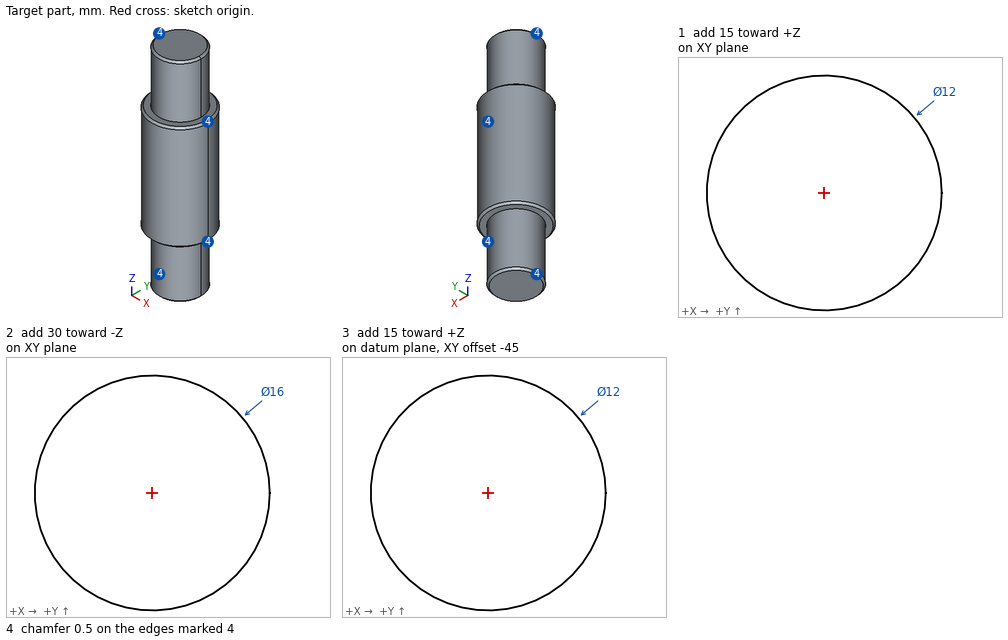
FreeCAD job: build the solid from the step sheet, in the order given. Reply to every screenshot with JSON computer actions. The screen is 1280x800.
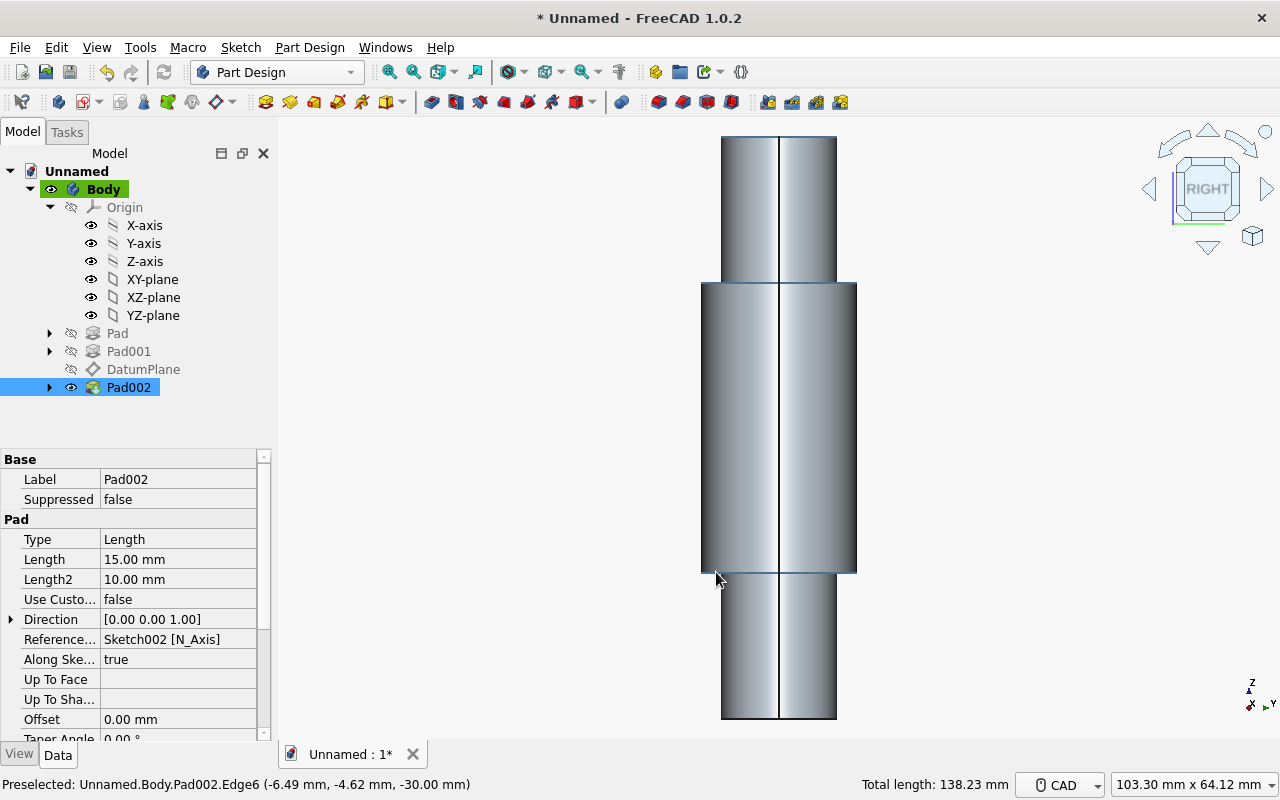
{"action": "key", "text": "5"}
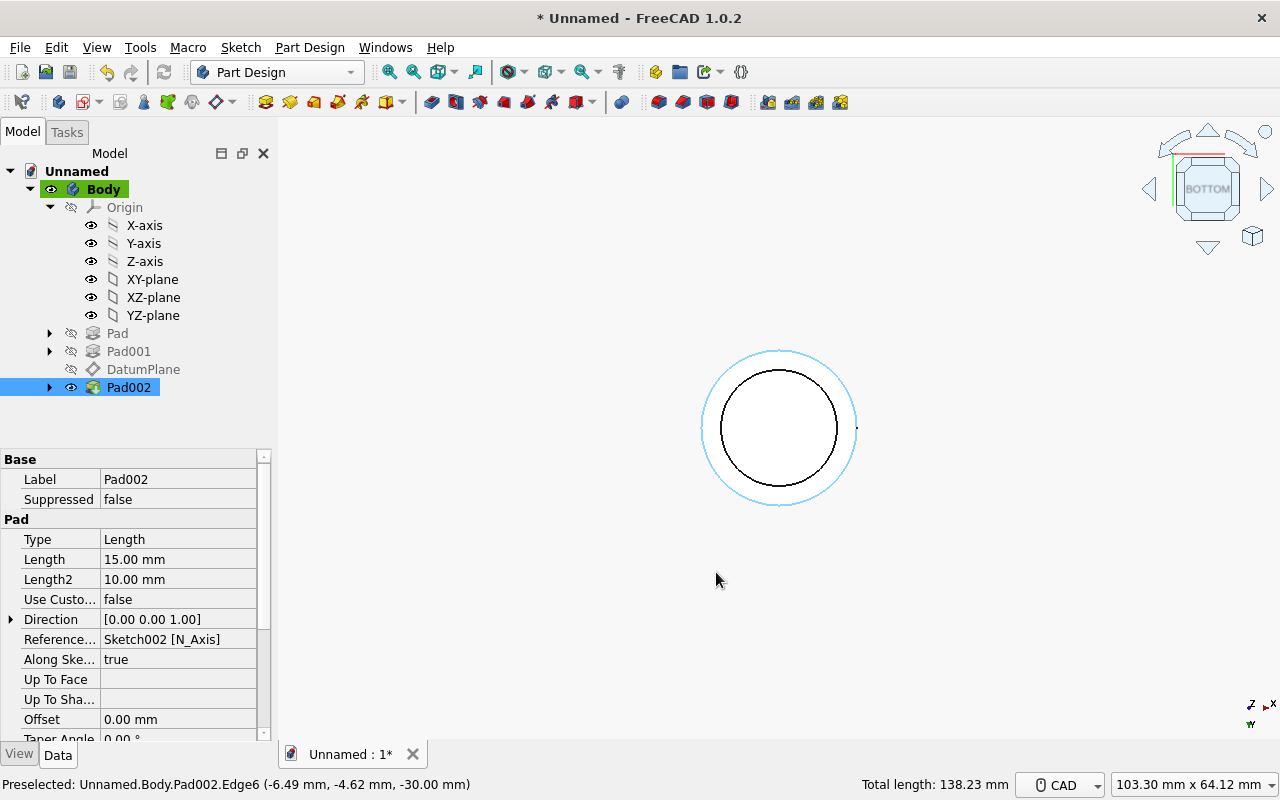
{"action": "left_click", "coordinate": [390, 72]}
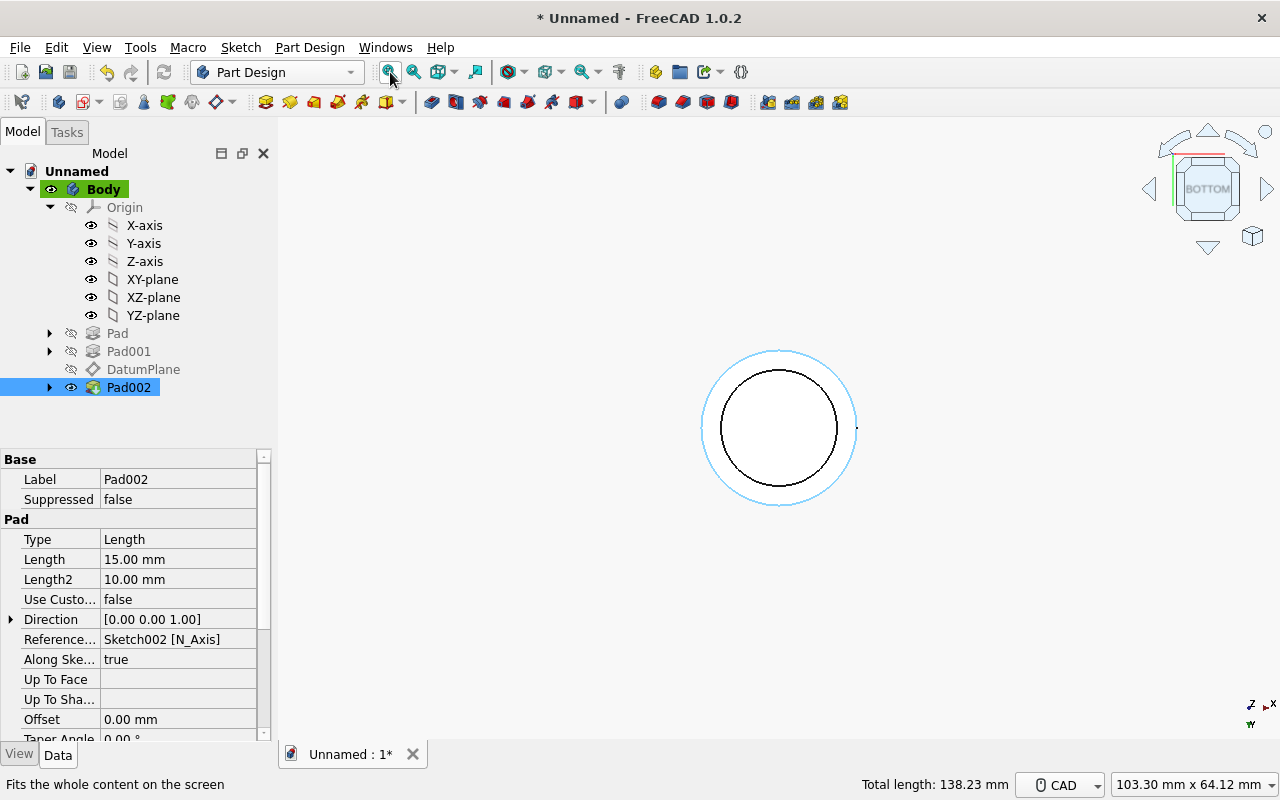
{"action": "left_click", "coordinate": [721, 427], "text": "ctrl"}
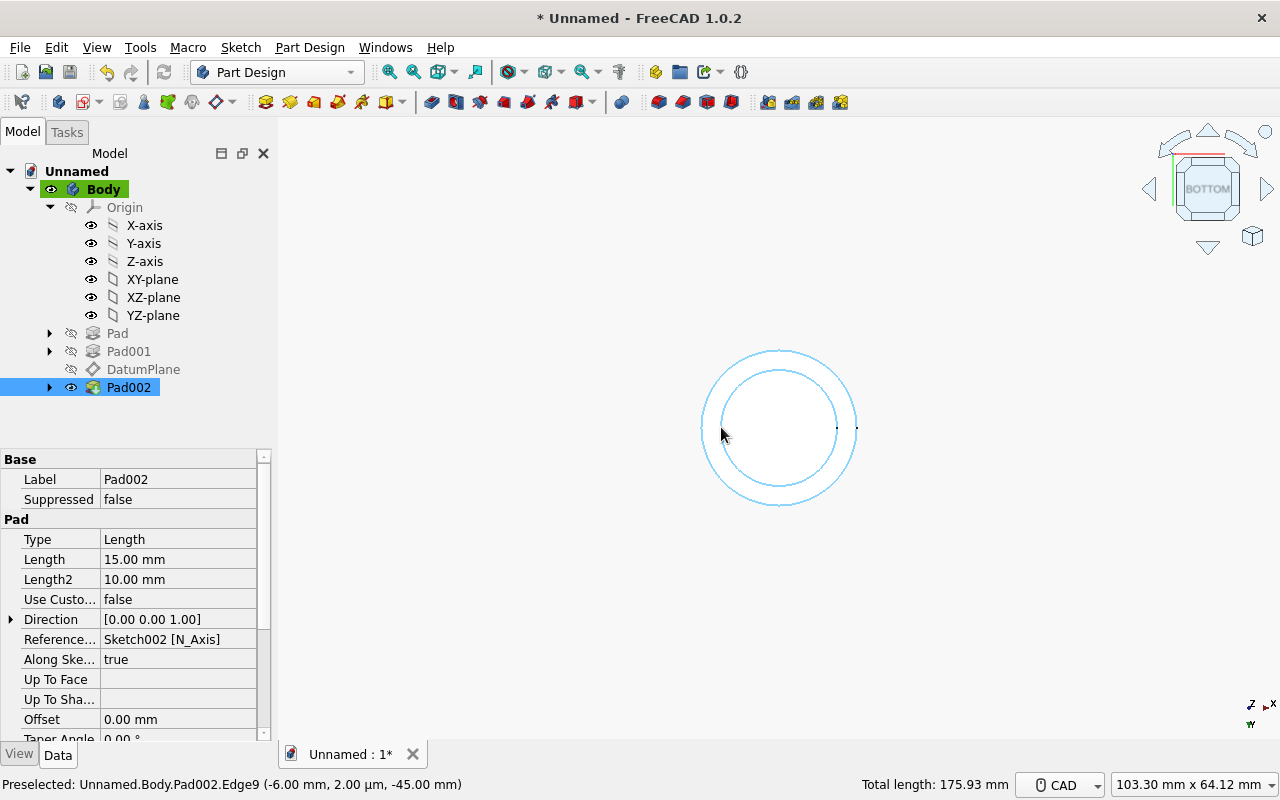
{"action": "left_click", "coordinate": [684, 102]}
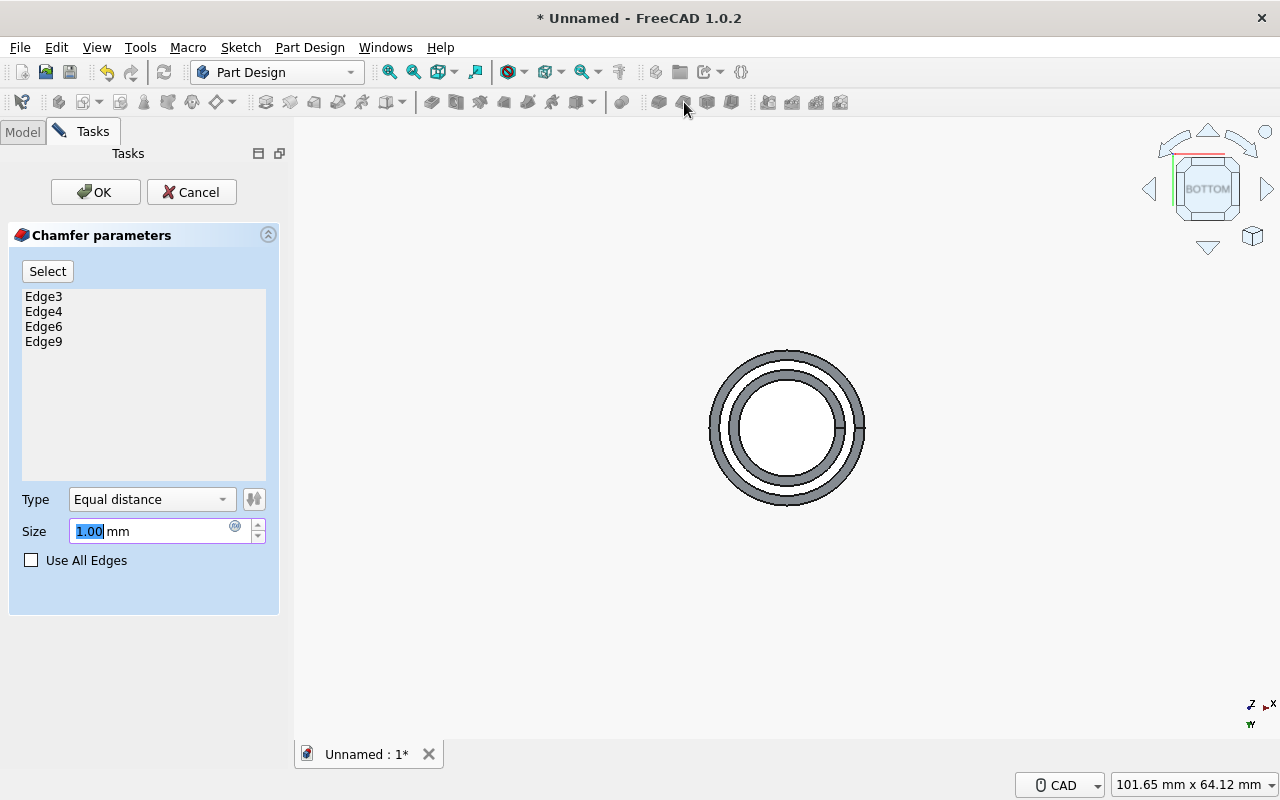
{"action": "type", "text": "0.5"}
{"action": "key", "text": "Tab"}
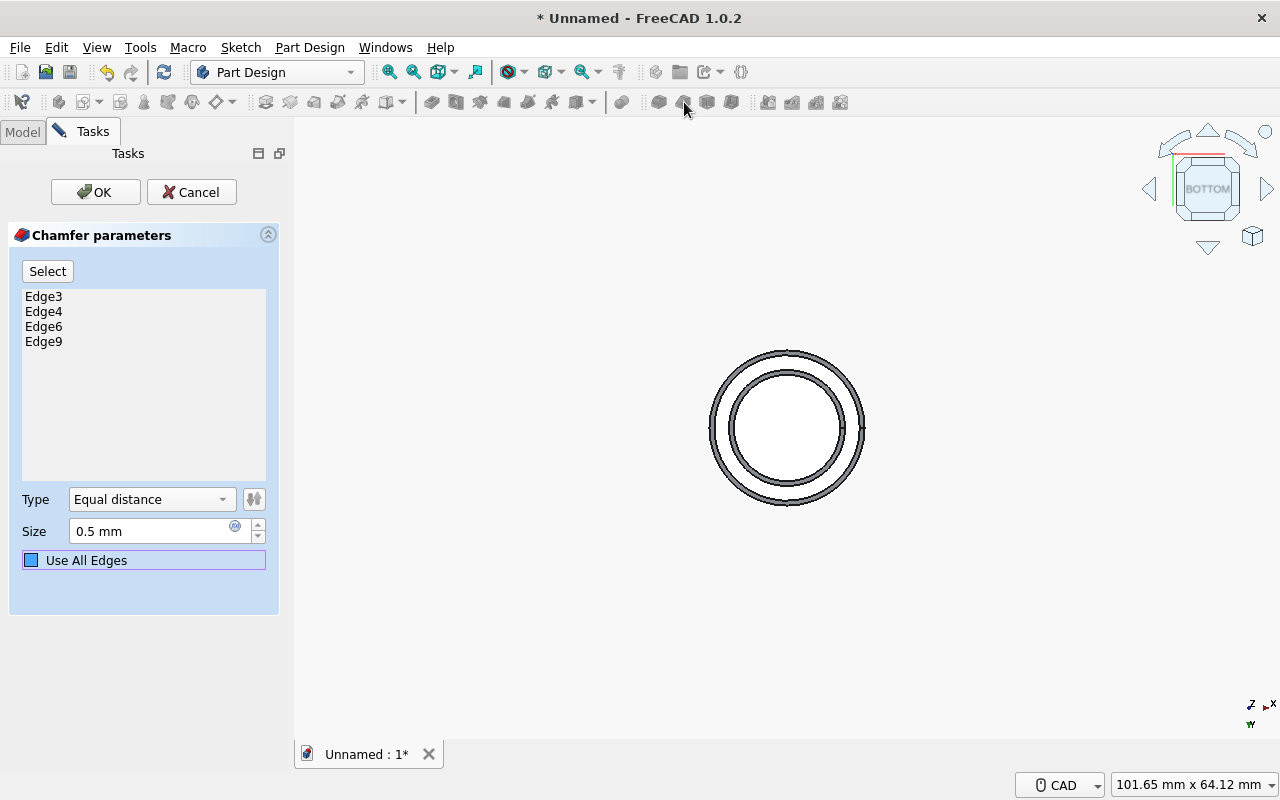
{"action": "left_click", "coordinate": [96, 192]}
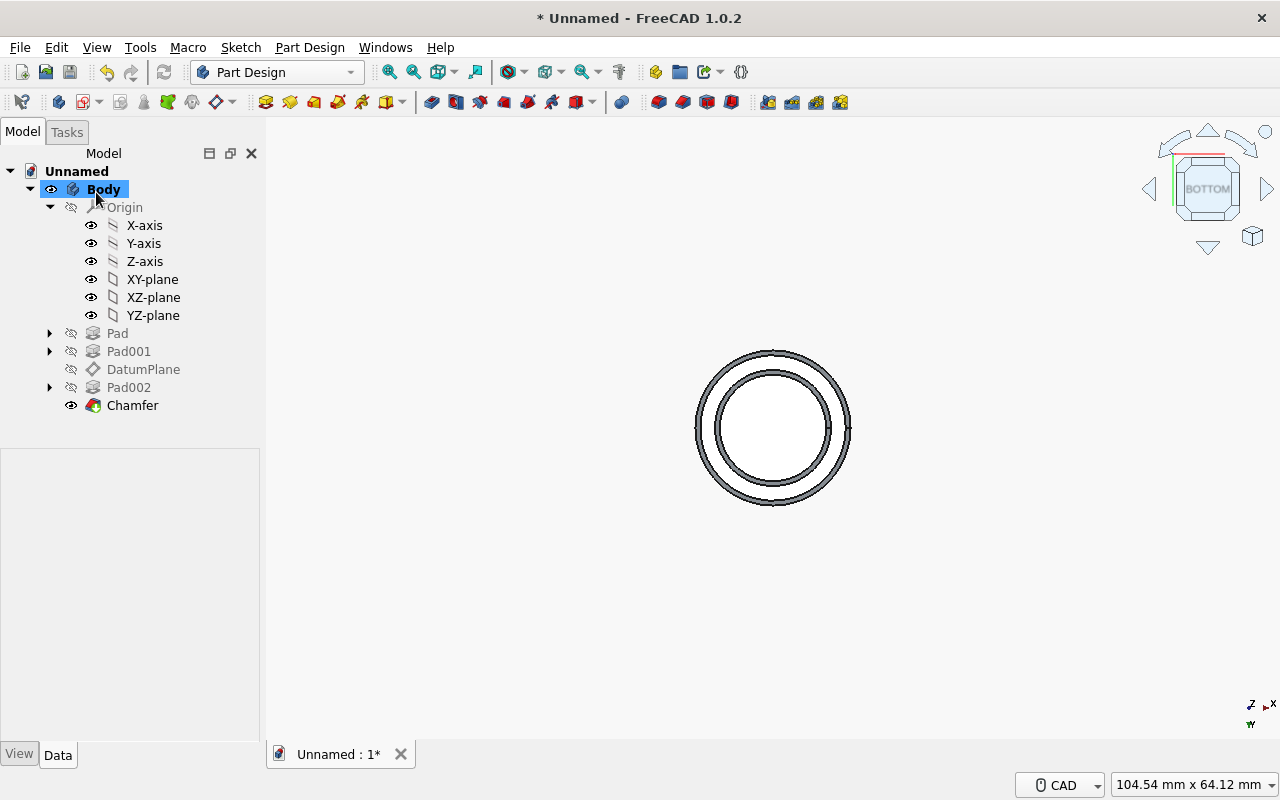
{"action": "key", "text": "0"}